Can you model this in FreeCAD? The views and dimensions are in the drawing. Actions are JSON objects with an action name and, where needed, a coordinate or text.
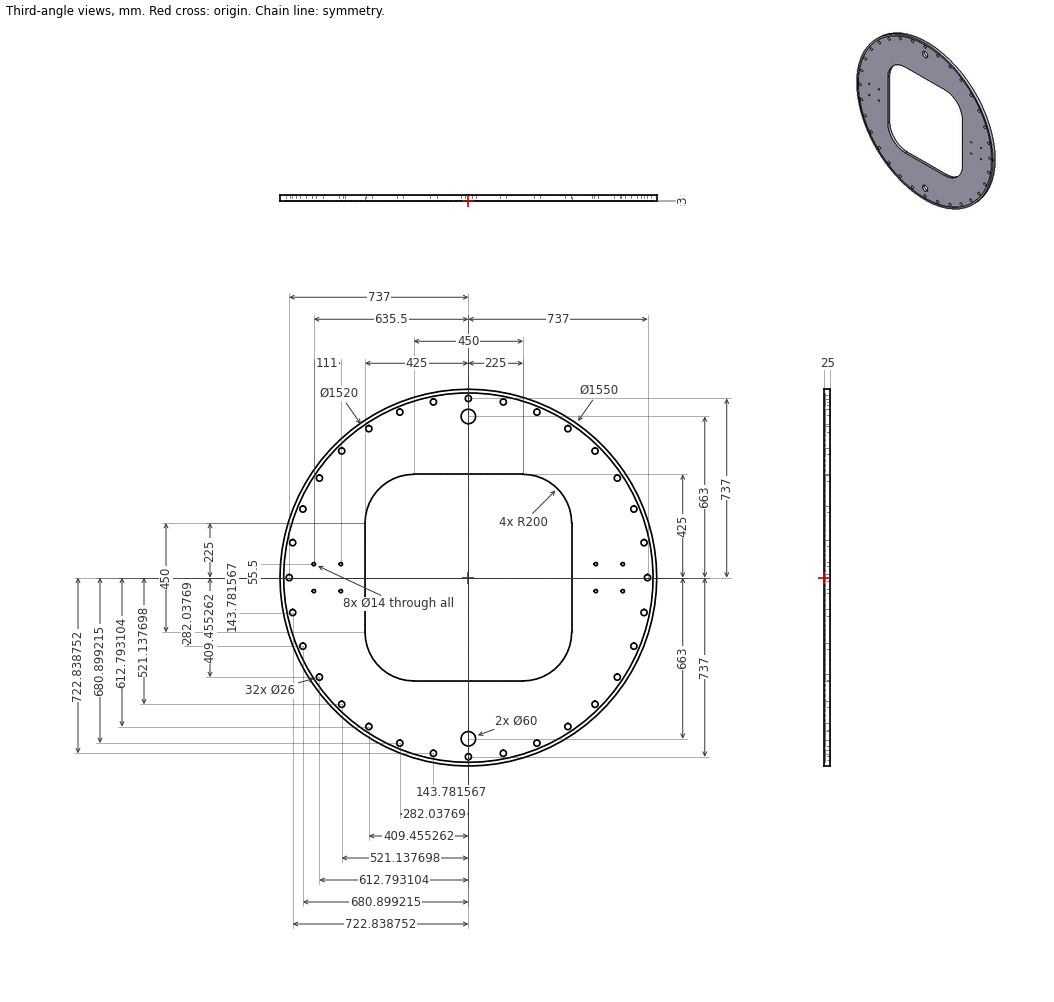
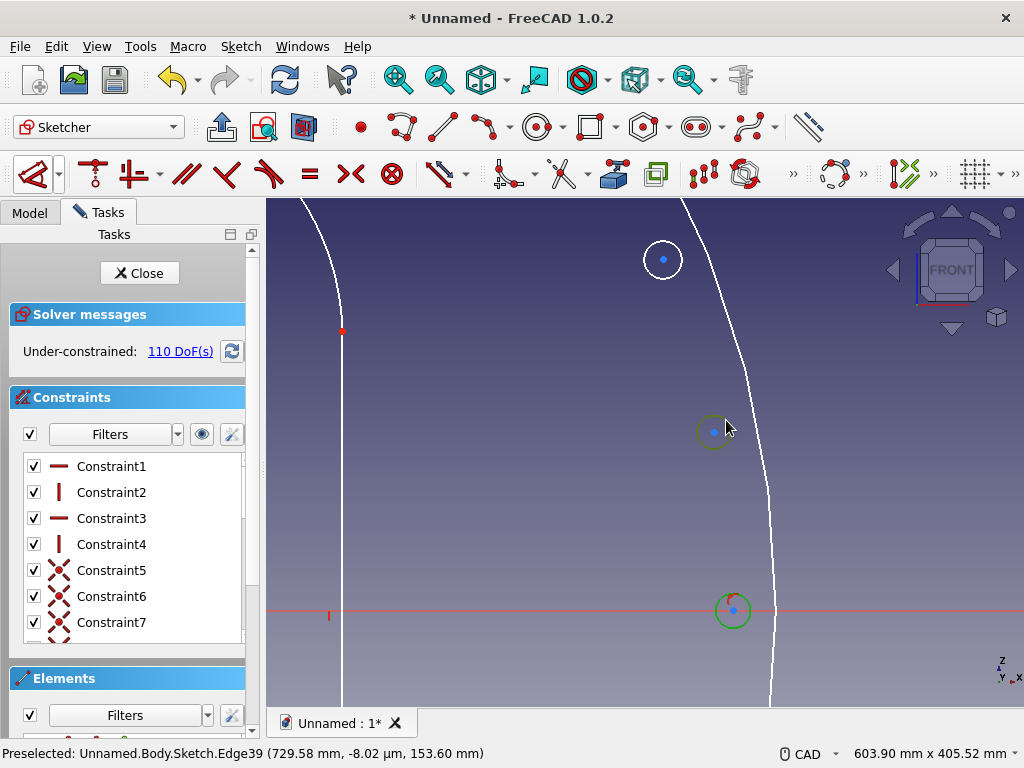
{"action": "left_click", "coordinate": [676, 247]}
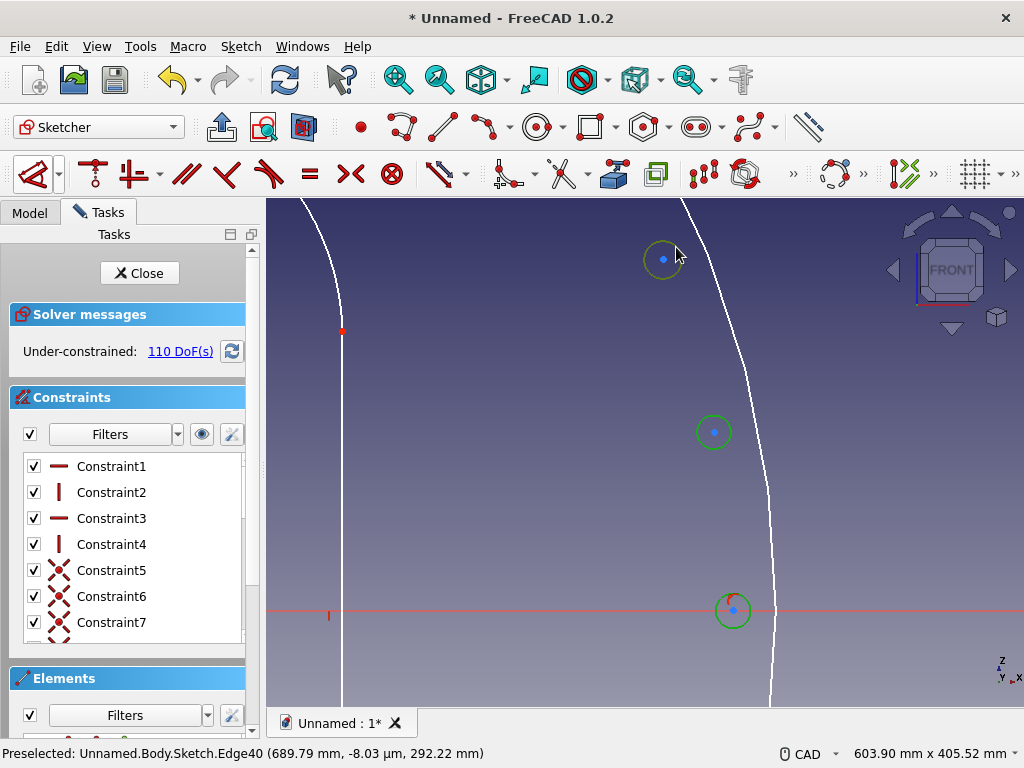
{"action": "scroll", "coordinate": [729, 421], "scroll_direction": "down", "scroll_amount": 9}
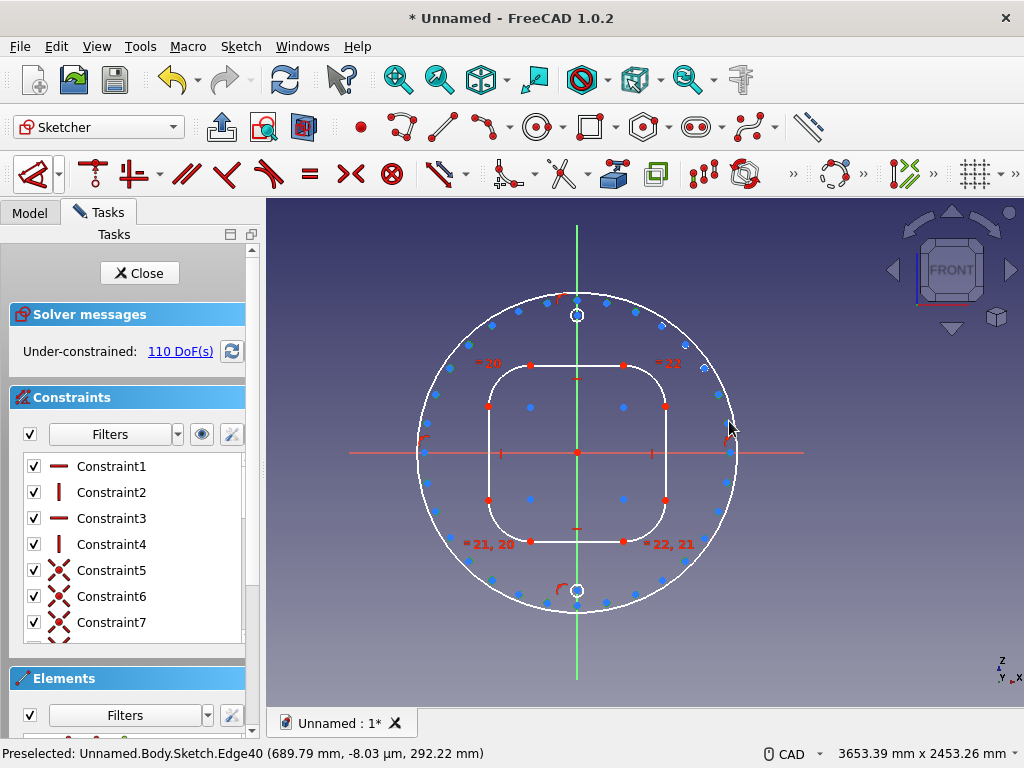
{"action": "scroll", "coordinate": [687, 343], "scroll_direction": "up", "scroll_amount": 8}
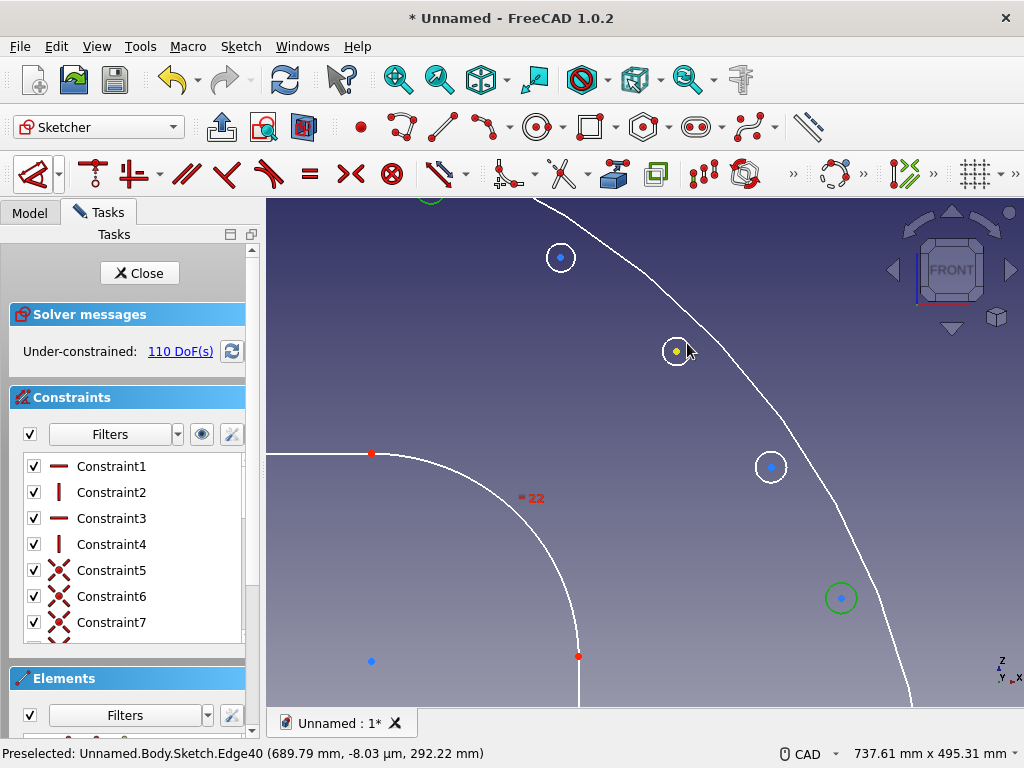
{"action": "left_click", "coordinate": [687, 342]}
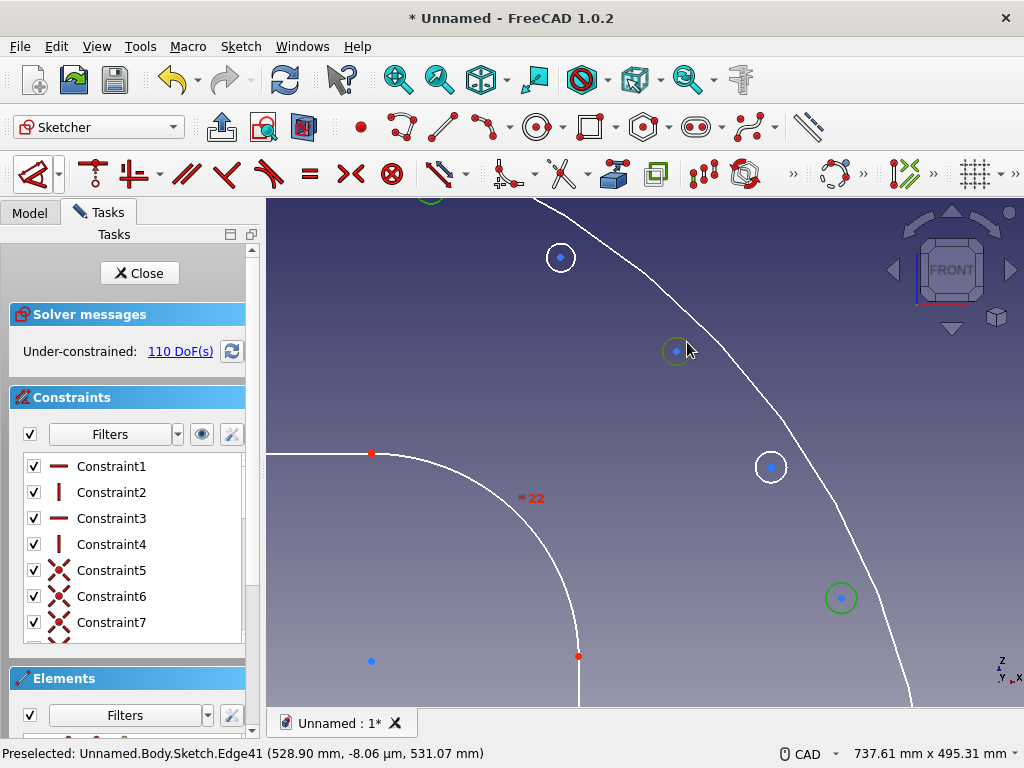
{"action": "left_click", "coordinate": [571, 248]}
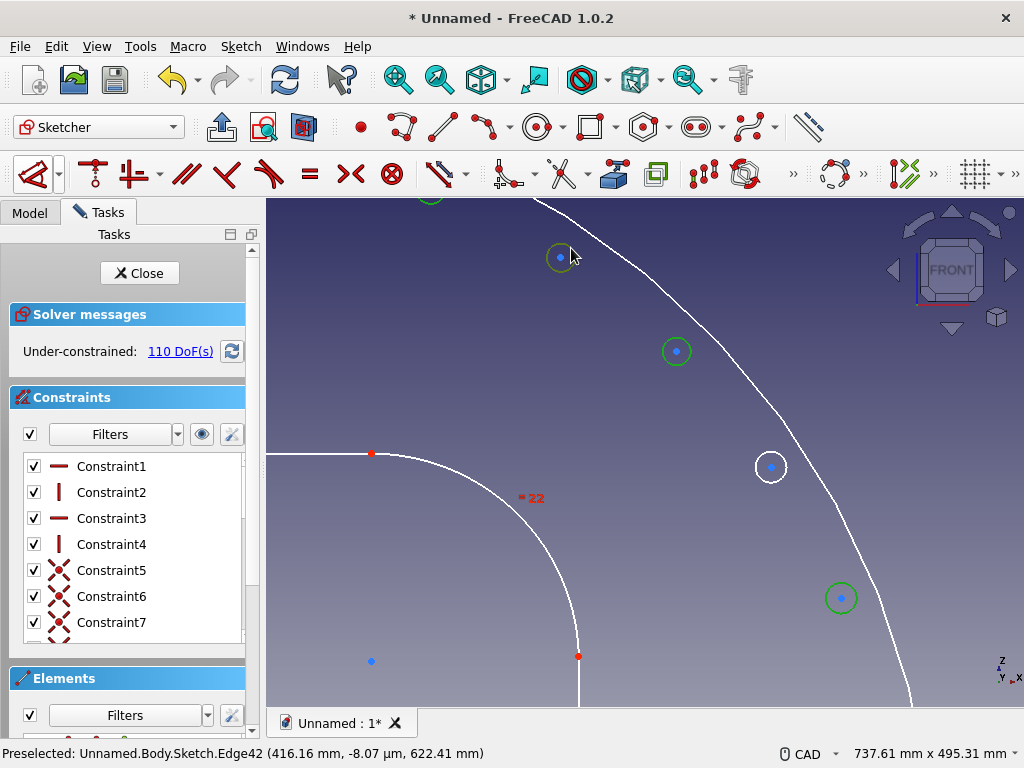
{"action": "left_click", "coordinate": [782, 456]}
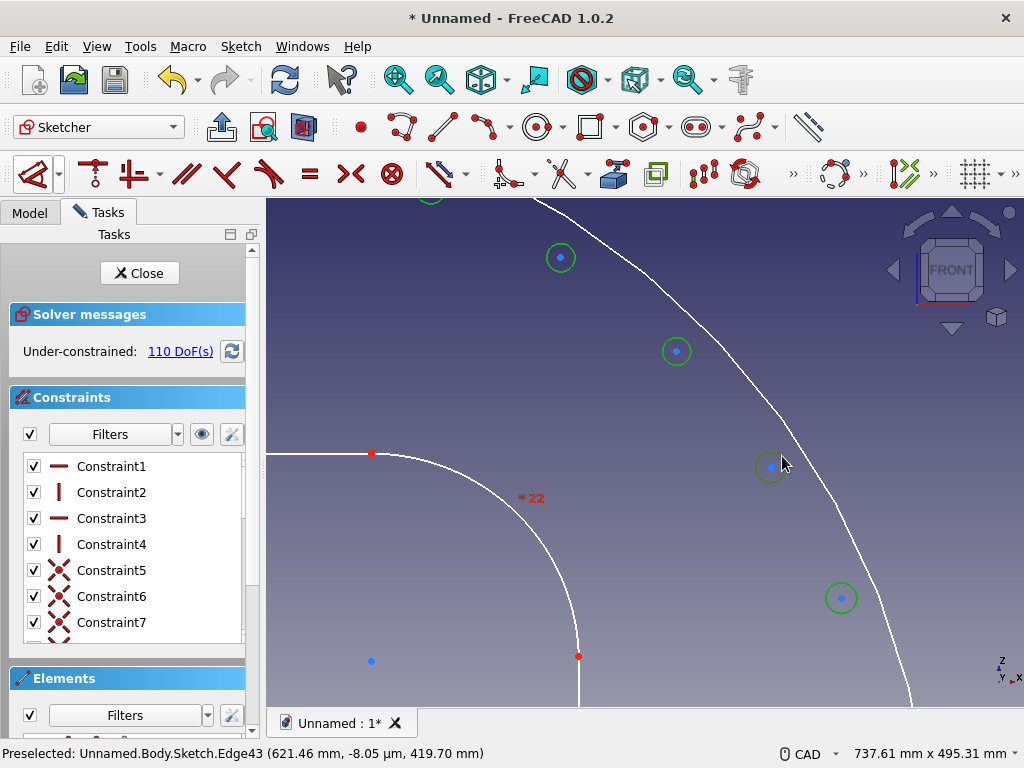
{"action": "left_click", "coordinate": [310, 174]}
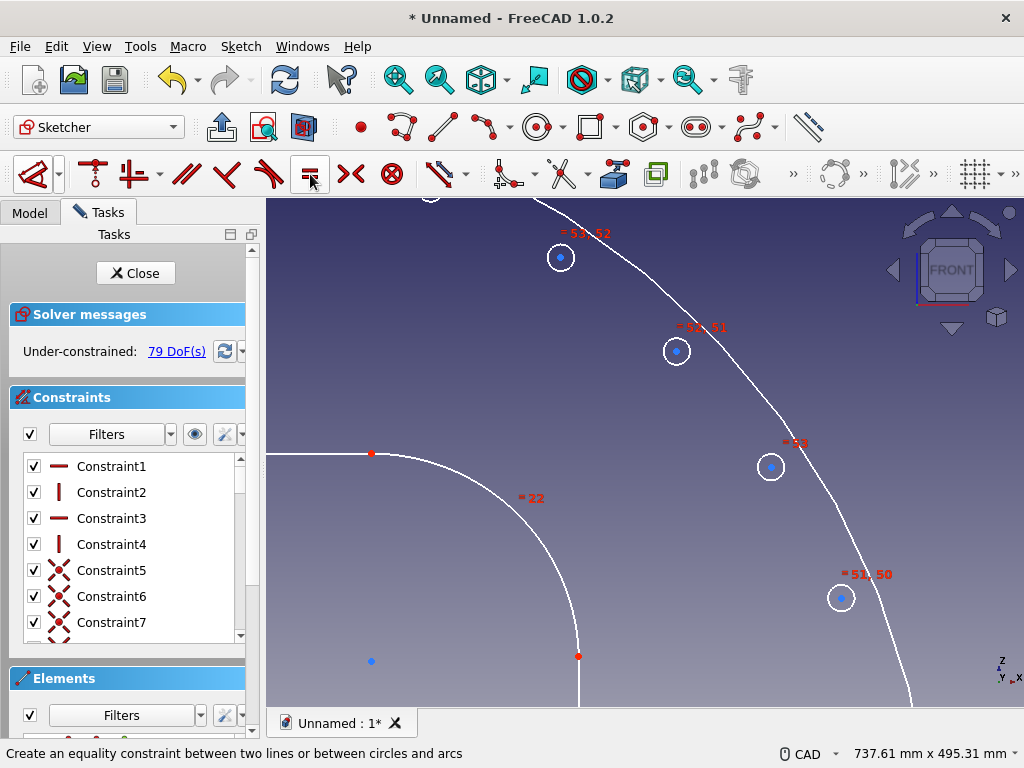
{"action": "scroll", "coordinate": [687, 343], "scroll_direction": "down", "scroll_amount": 8}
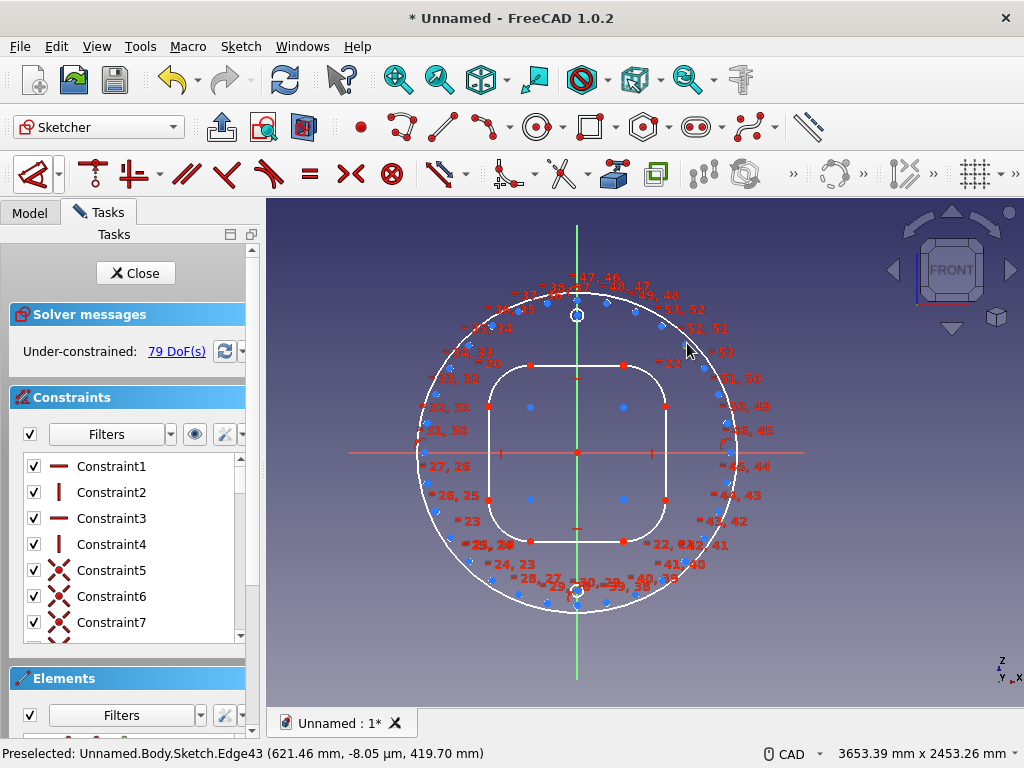
{"action": "scroll", "coordinate": [582, 586], "scroll_direction": "up", "scroll_amount": 6}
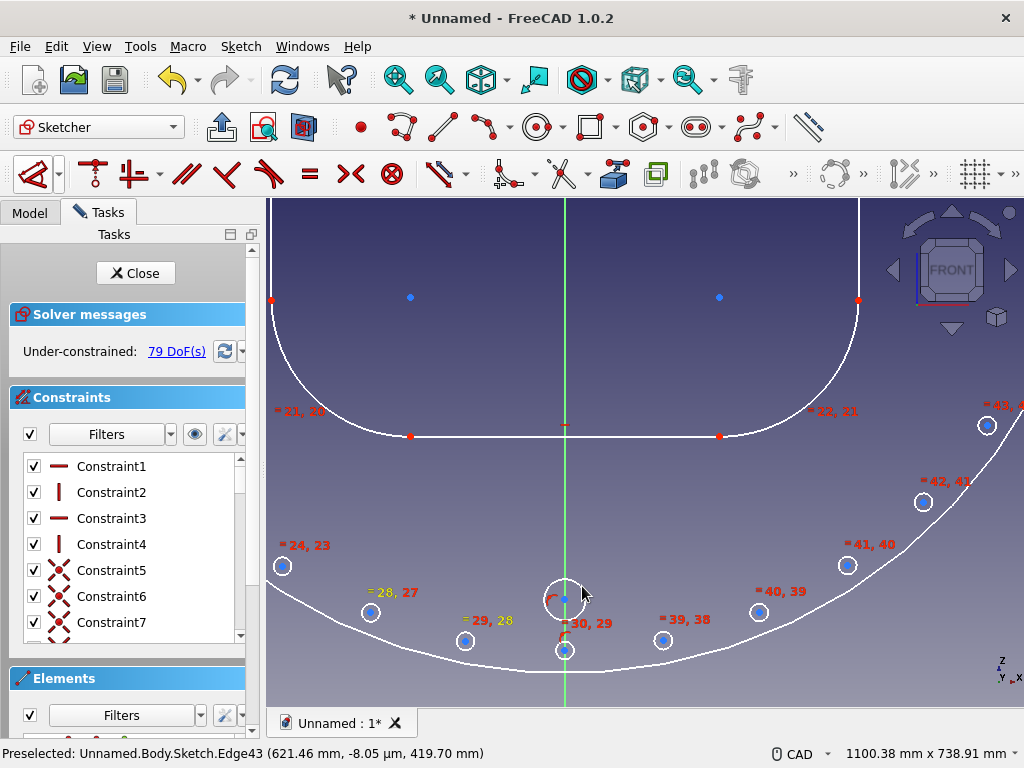
{"action": "left_click", "coordinate": [579, 585]}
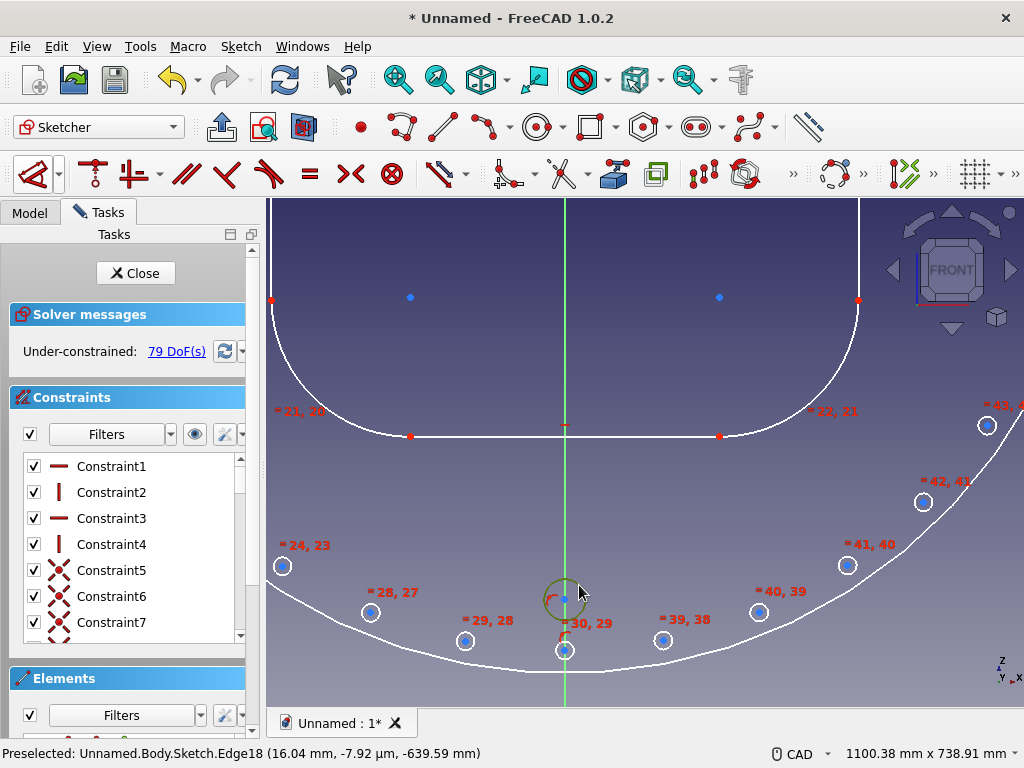
{"action": "scroll", "coordinate": [581, 586], "scroll_direction": "down", "scroll_amount": 6}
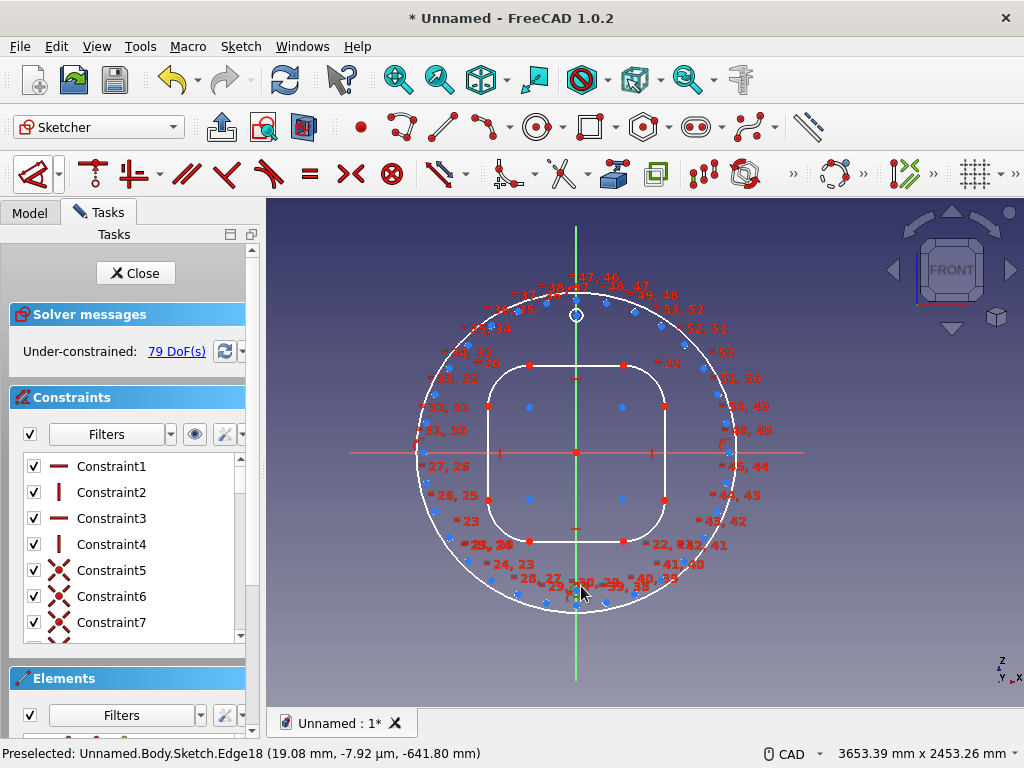
{"action": "scroll", "coordinate": [581, 311], "scroll_direction": "up", "scroll_amount": 6}